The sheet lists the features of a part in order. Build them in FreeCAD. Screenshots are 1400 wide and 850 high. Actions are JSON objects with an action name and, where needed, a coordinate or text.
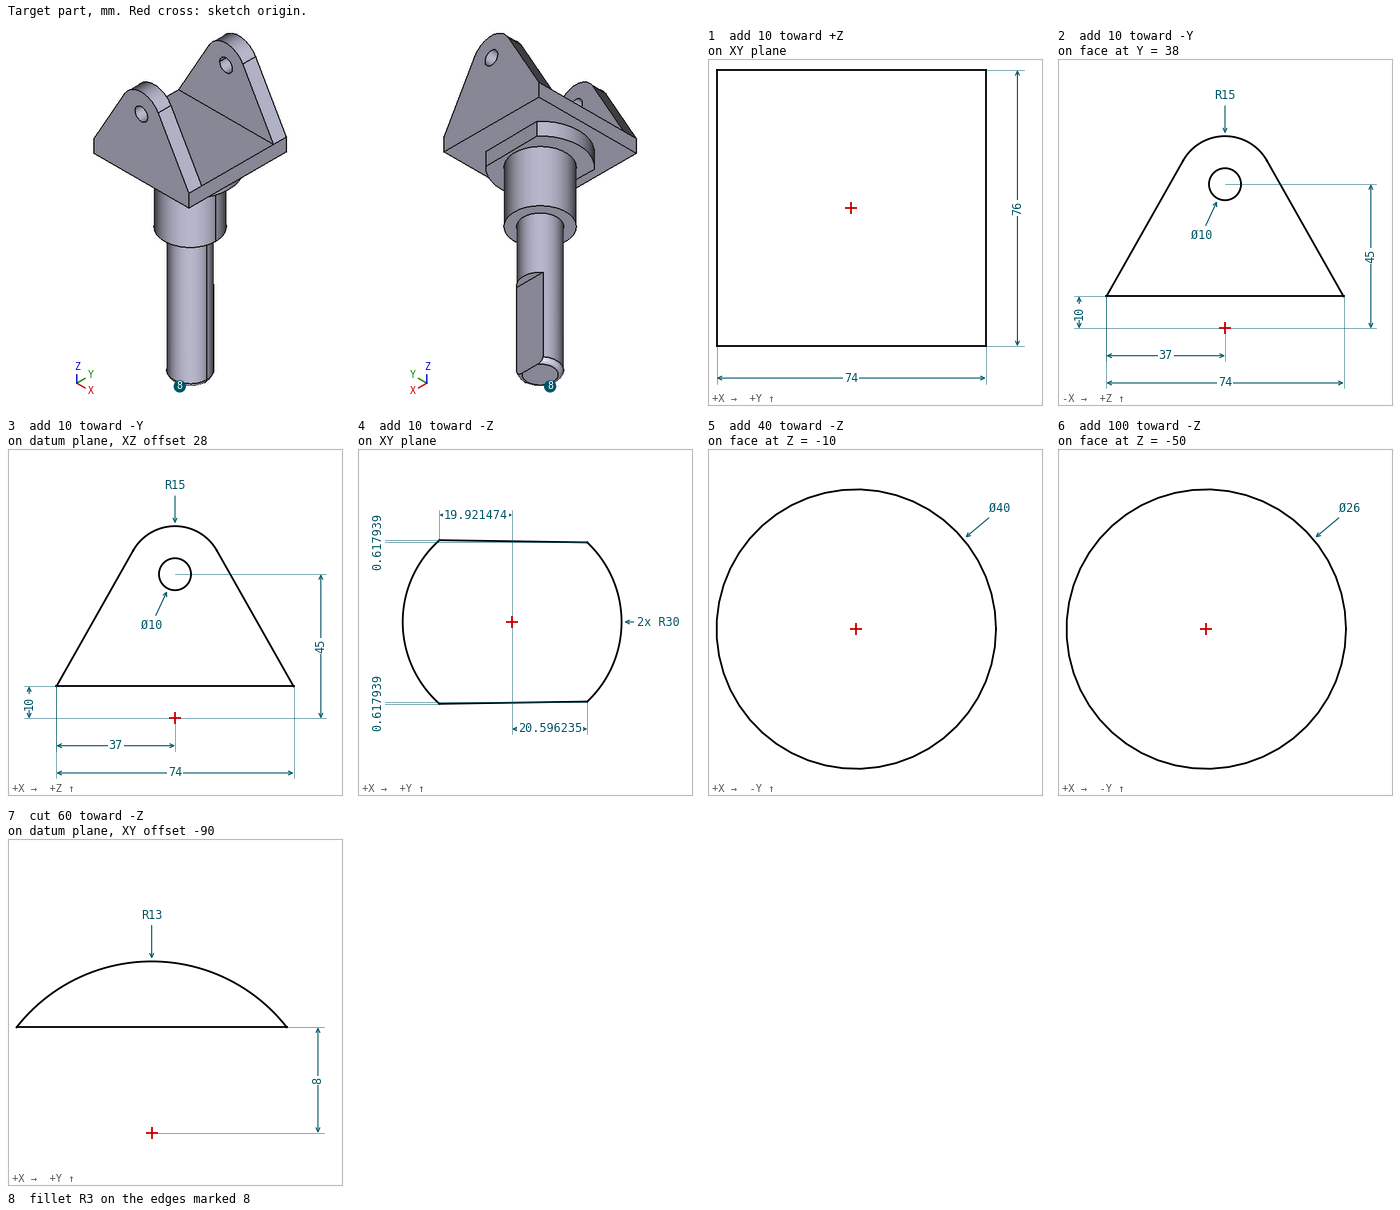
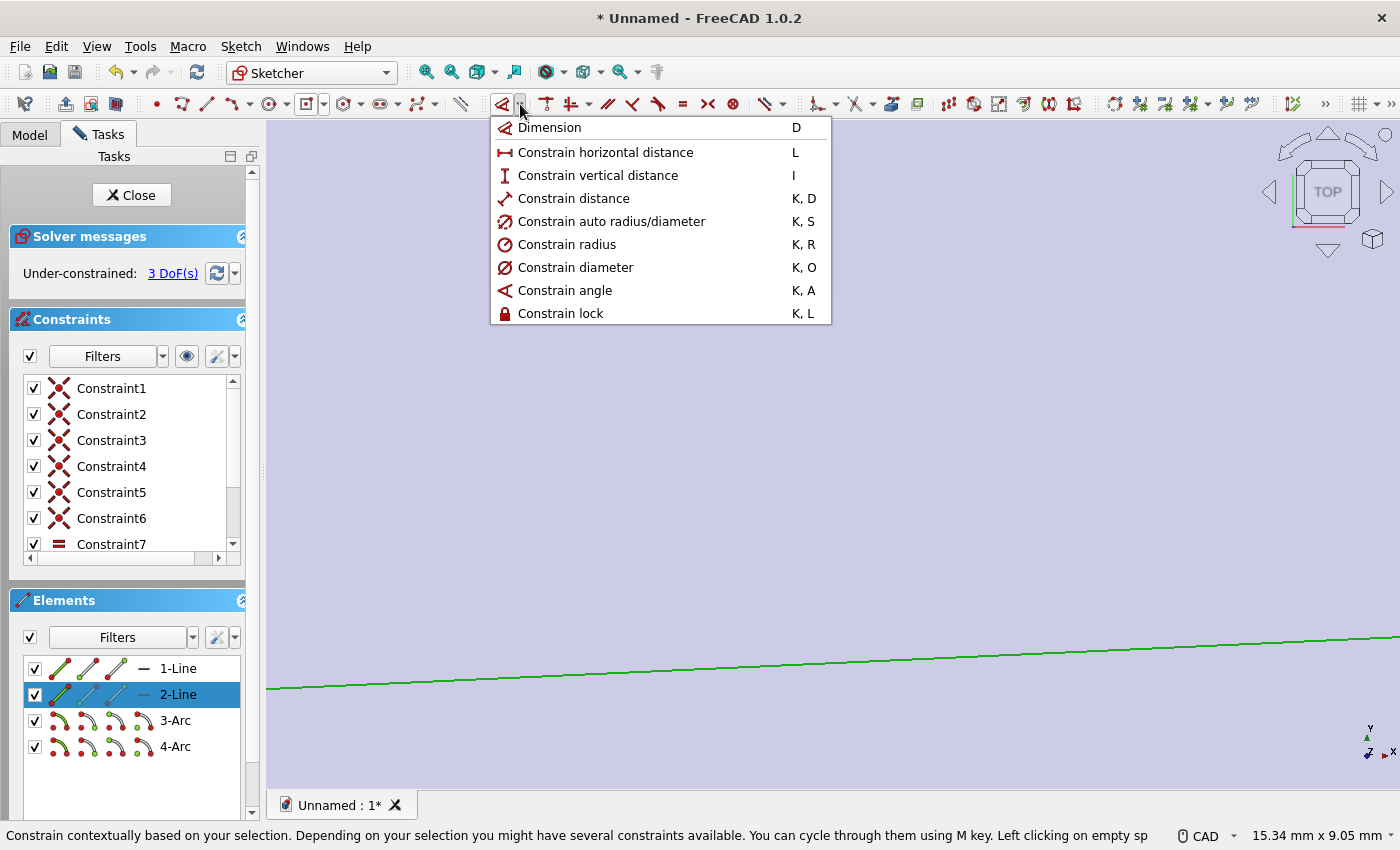
{"action": "left_click", "coordinate": [661, 176]}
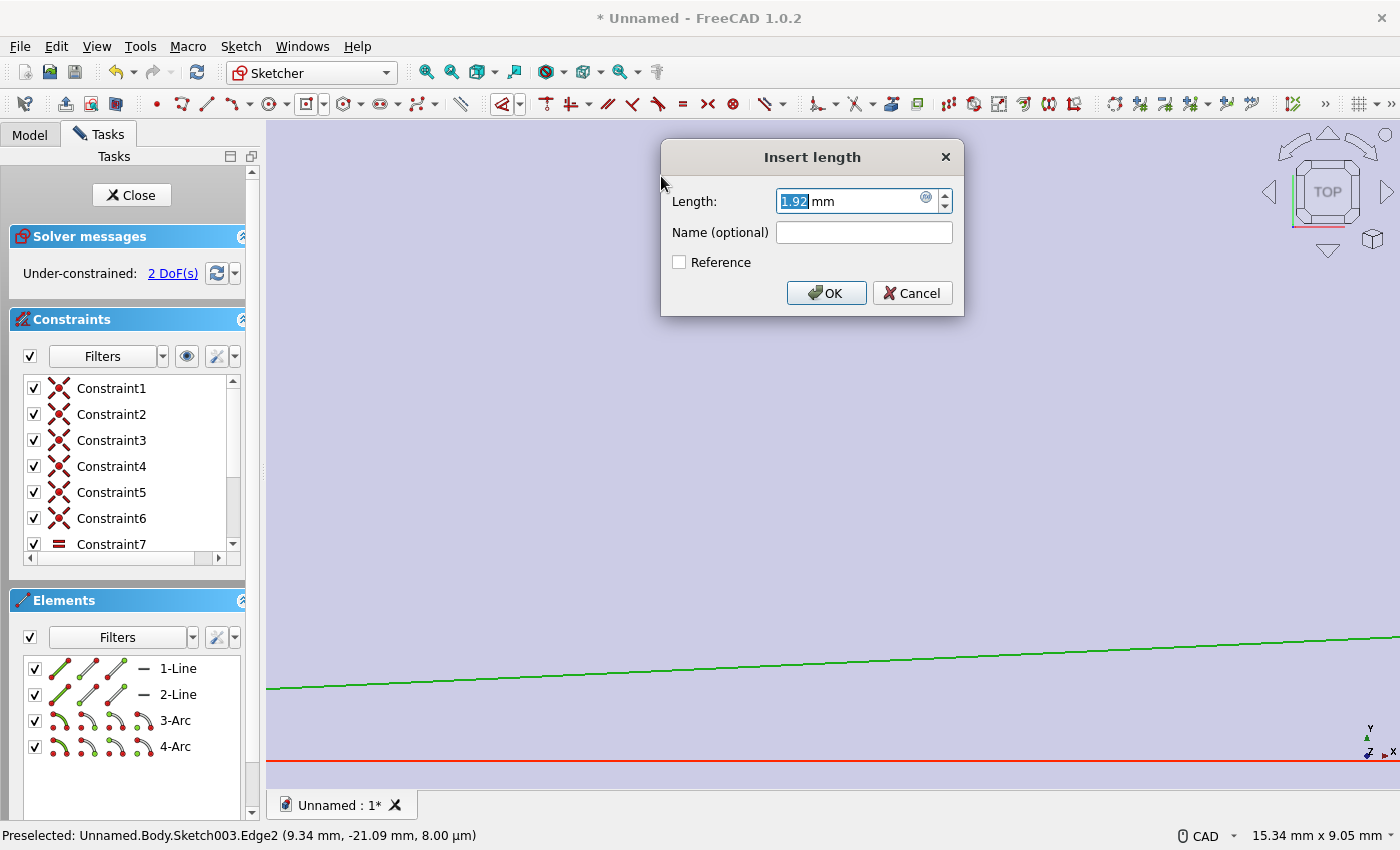
{"action": "type", "text": "0.617939"}
{"action": "key", "text": "Return"}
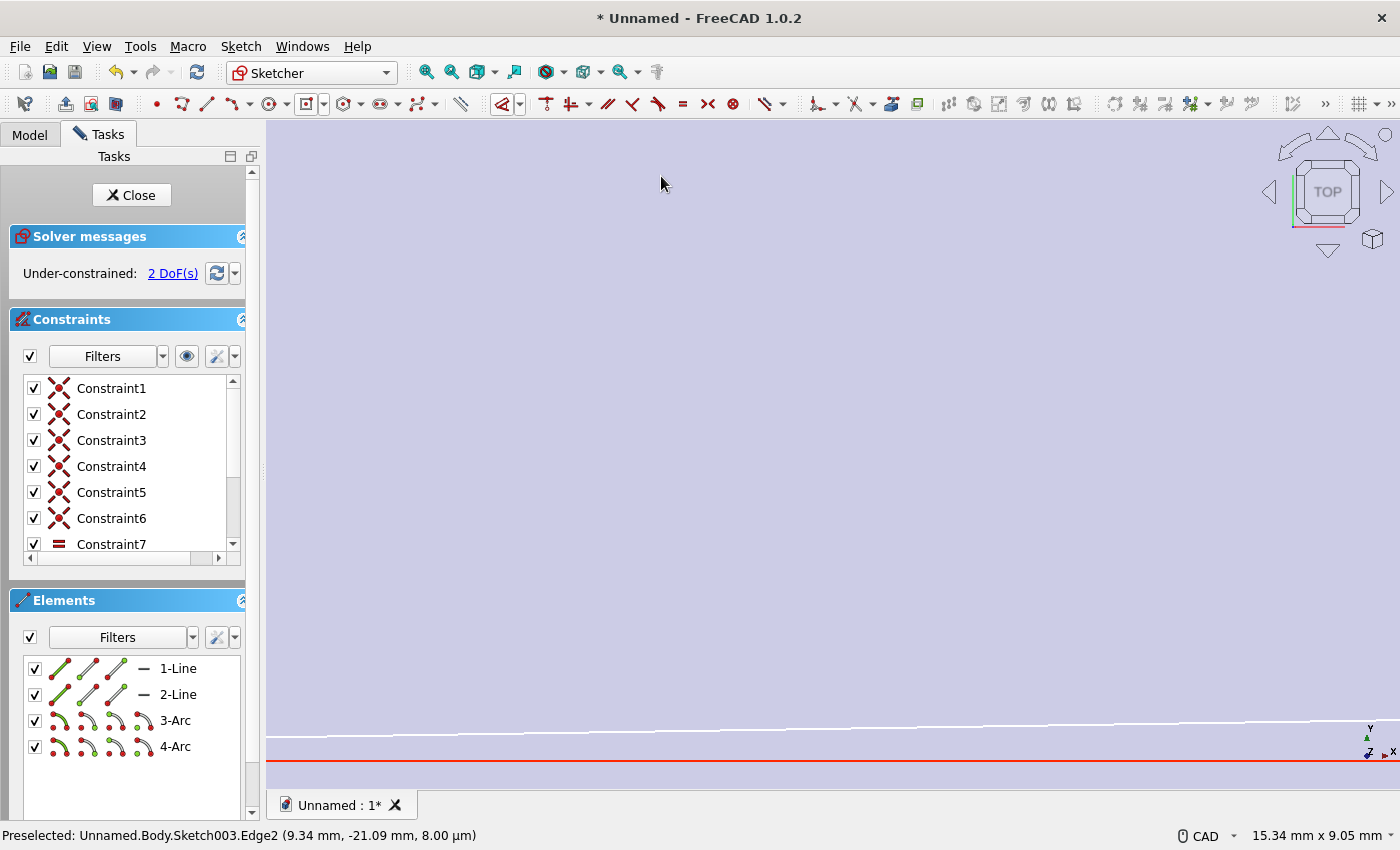
{"action": "scroll", "coordinate": [859, 666], "scroll_direction": "down", "scroll_amount": 10}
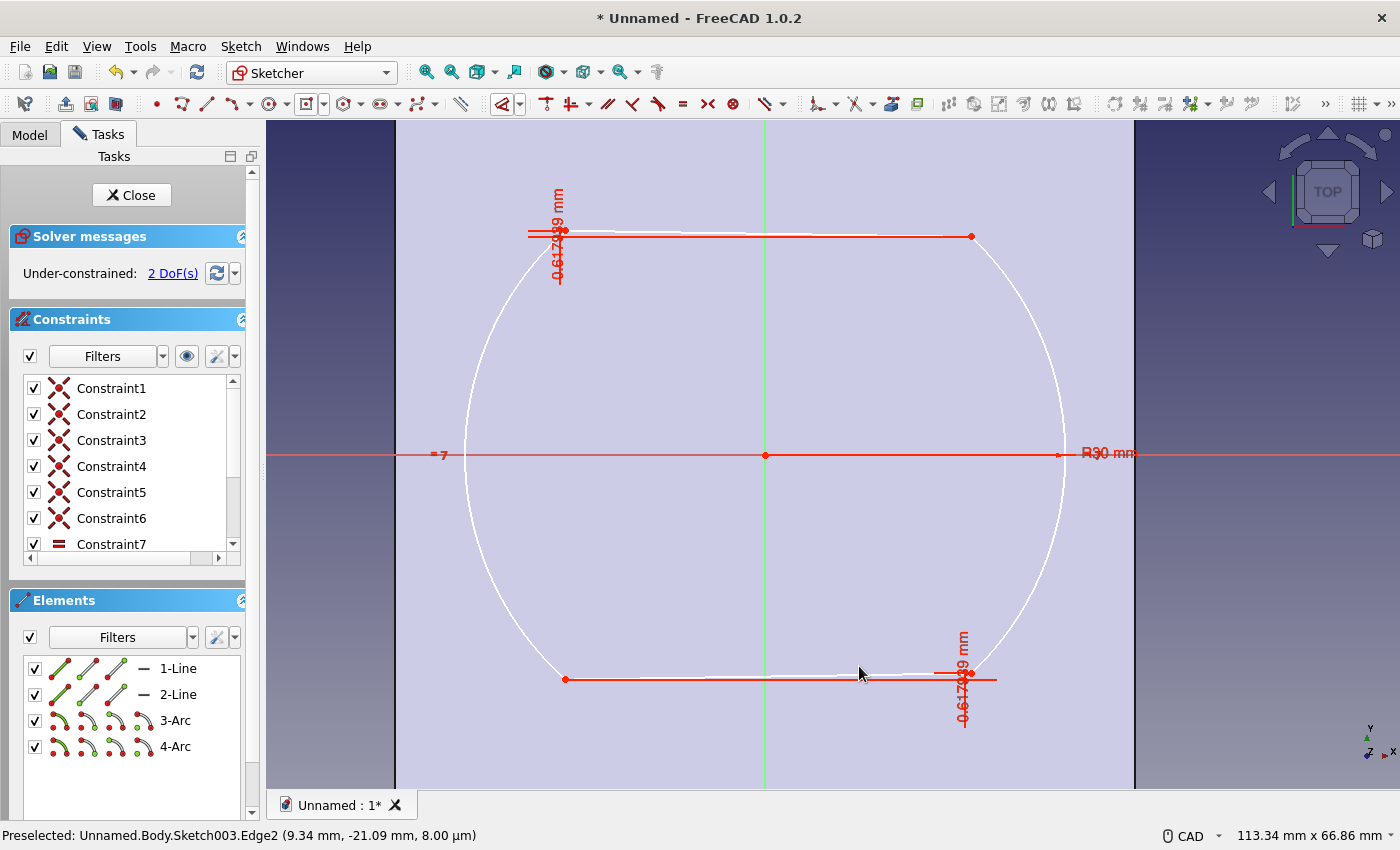
{"action": "left_click", "coordinate": [566, 231]}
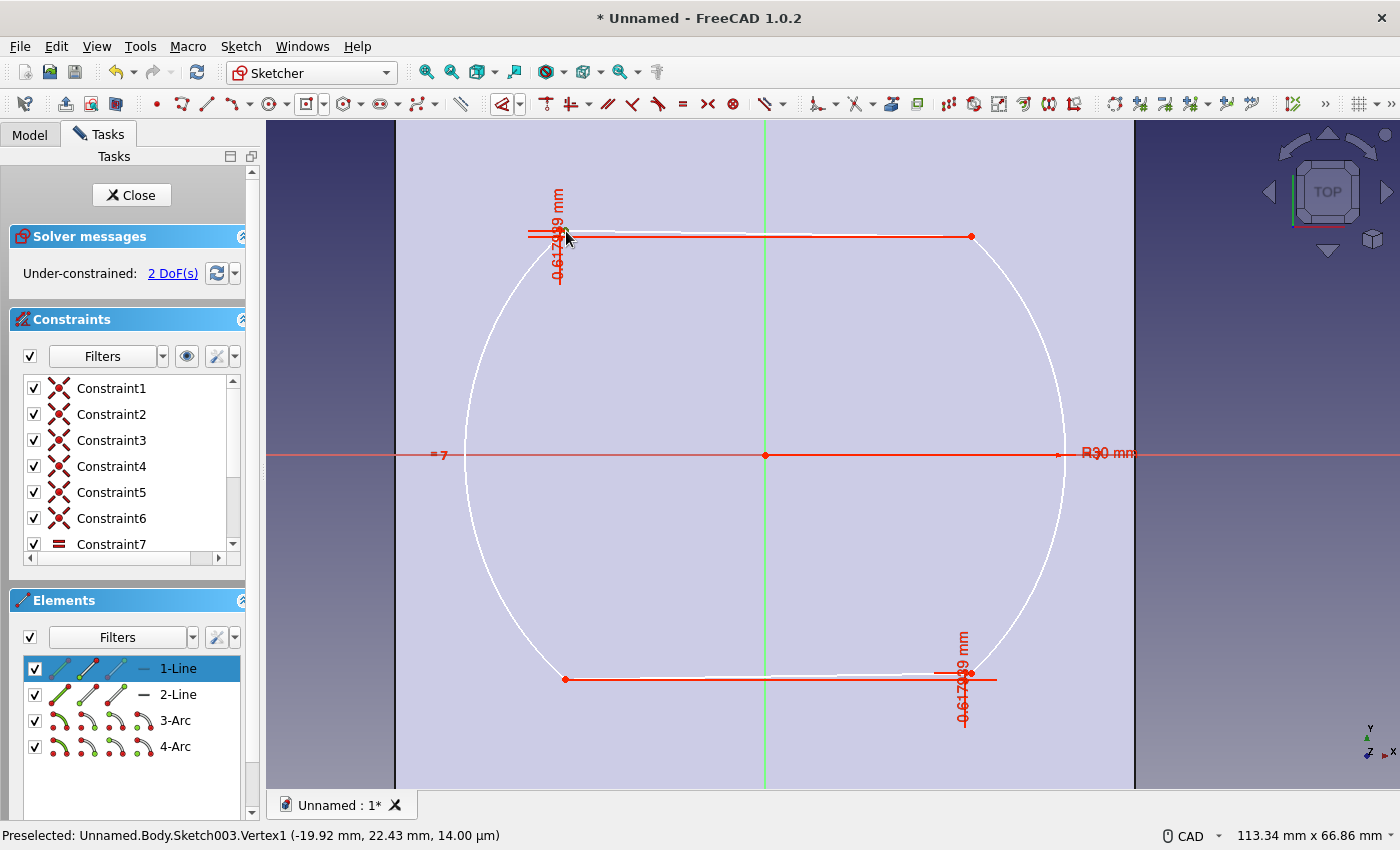
{"action": "left_click", "coordinate": [520, 104]}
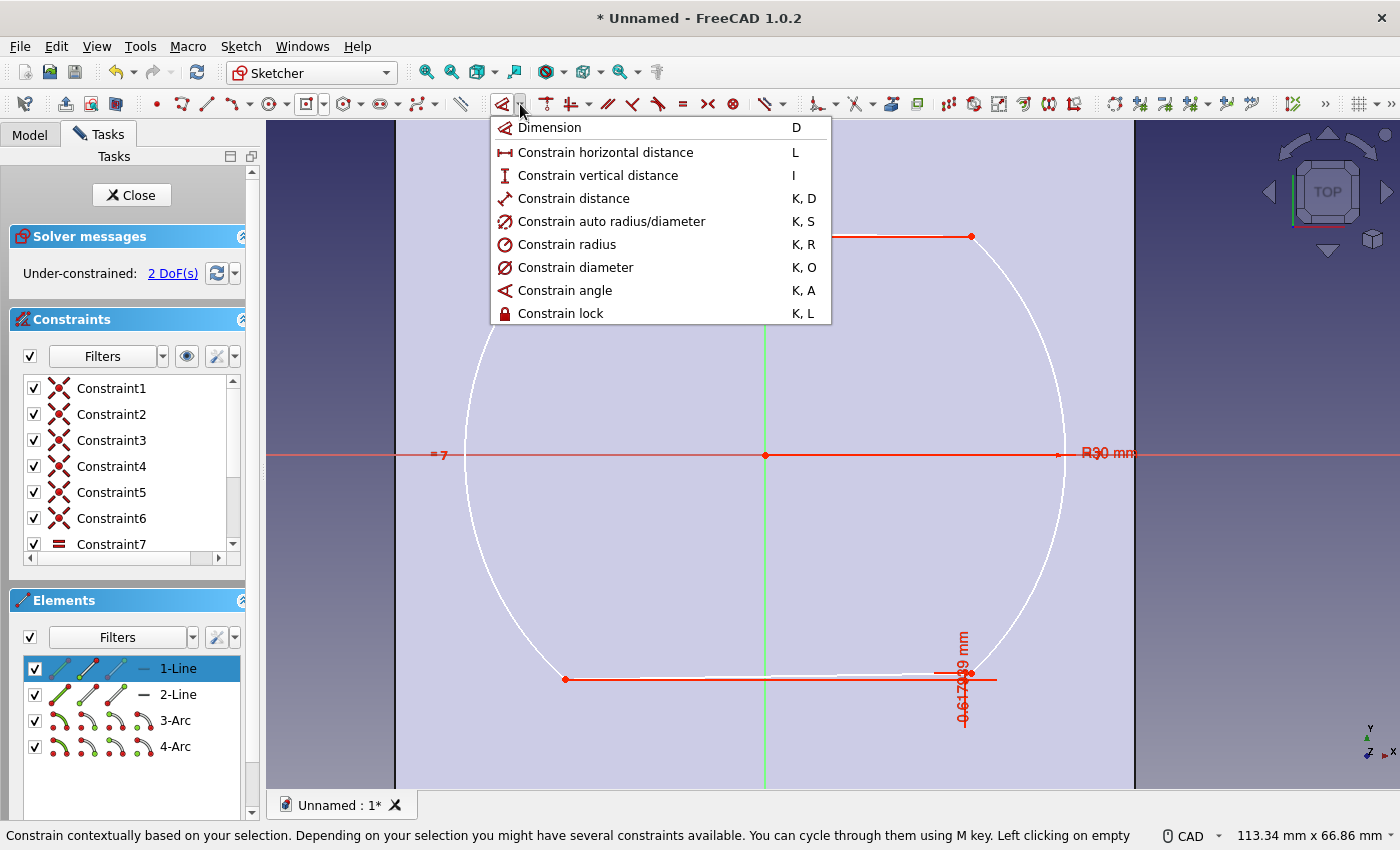
{"action": "left_click", "coordinate": [661, 152]}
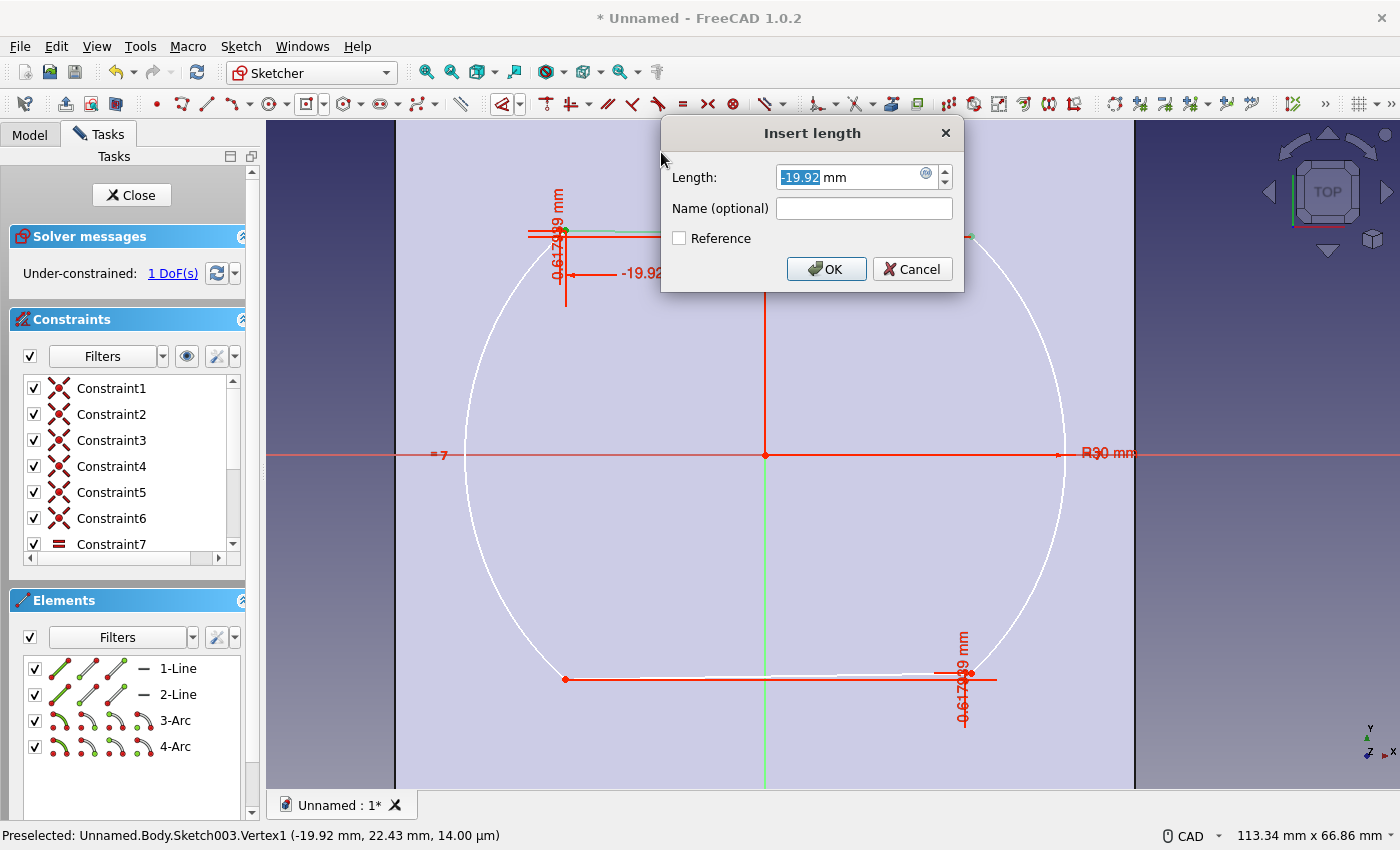
{"action": "type", "text": "-19.921474"}
{"action": "key", "text": "Return"}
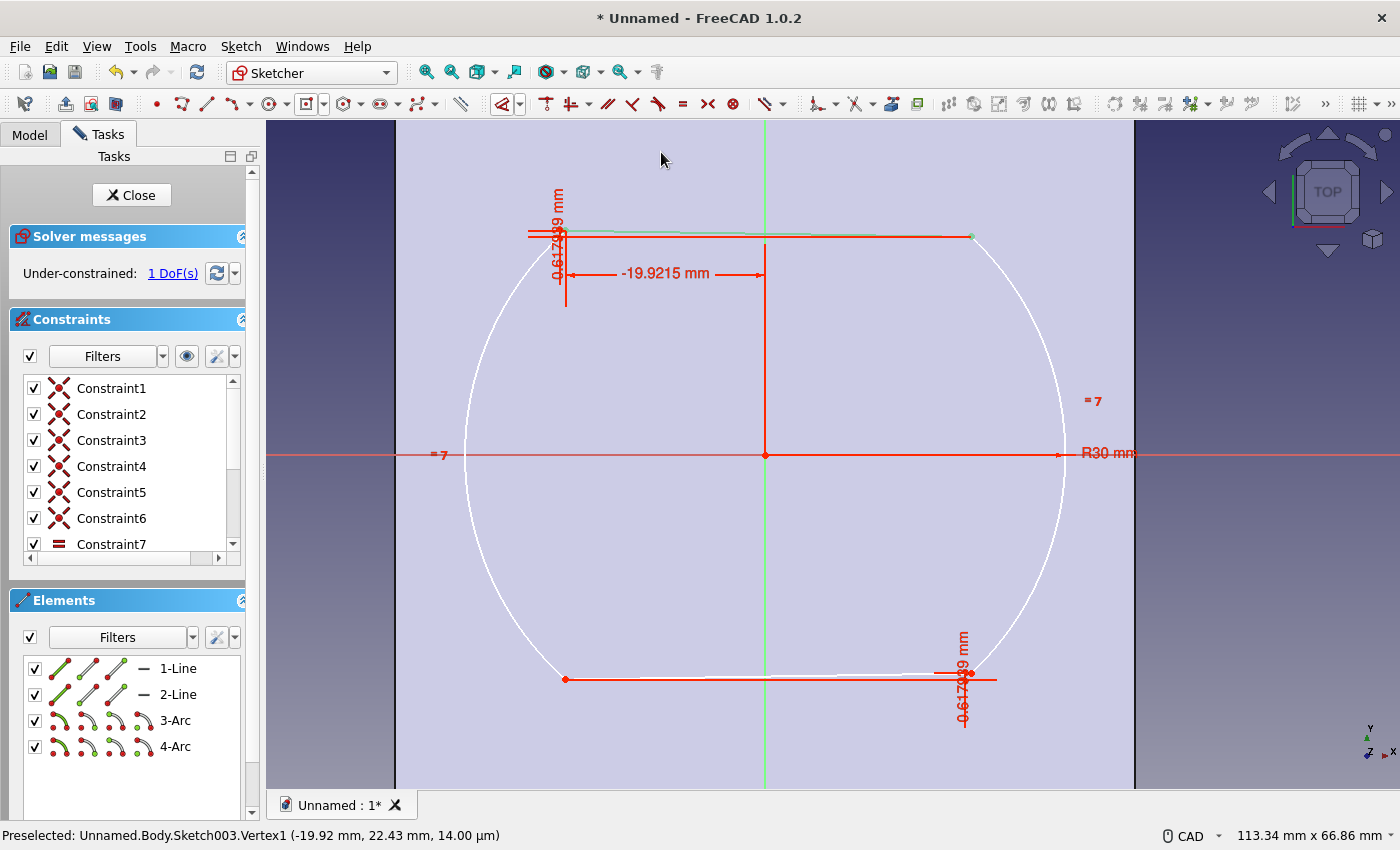
{"action": "left_click", "coordinate": [971, 673]}